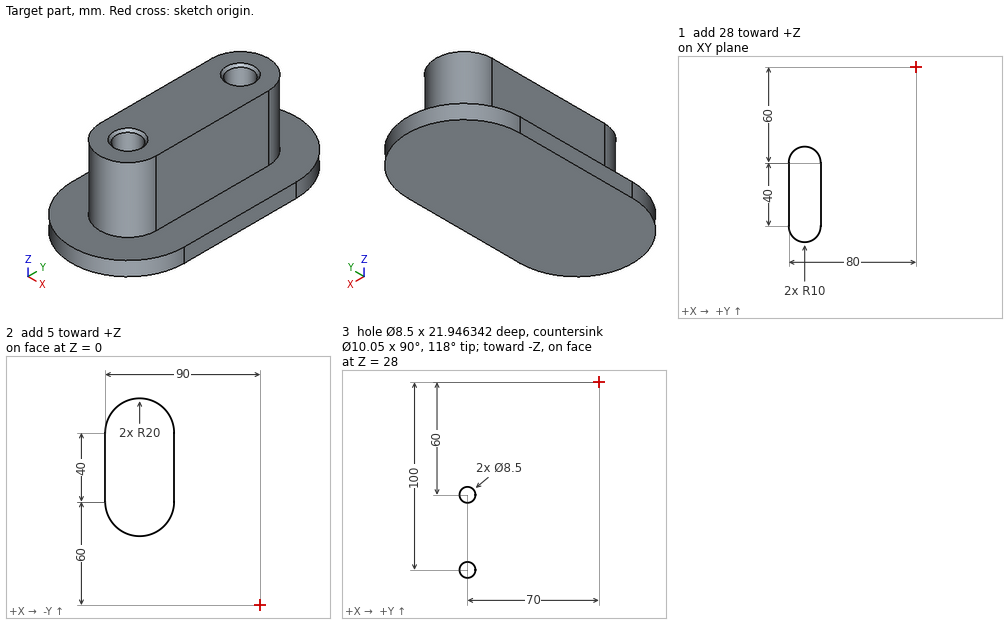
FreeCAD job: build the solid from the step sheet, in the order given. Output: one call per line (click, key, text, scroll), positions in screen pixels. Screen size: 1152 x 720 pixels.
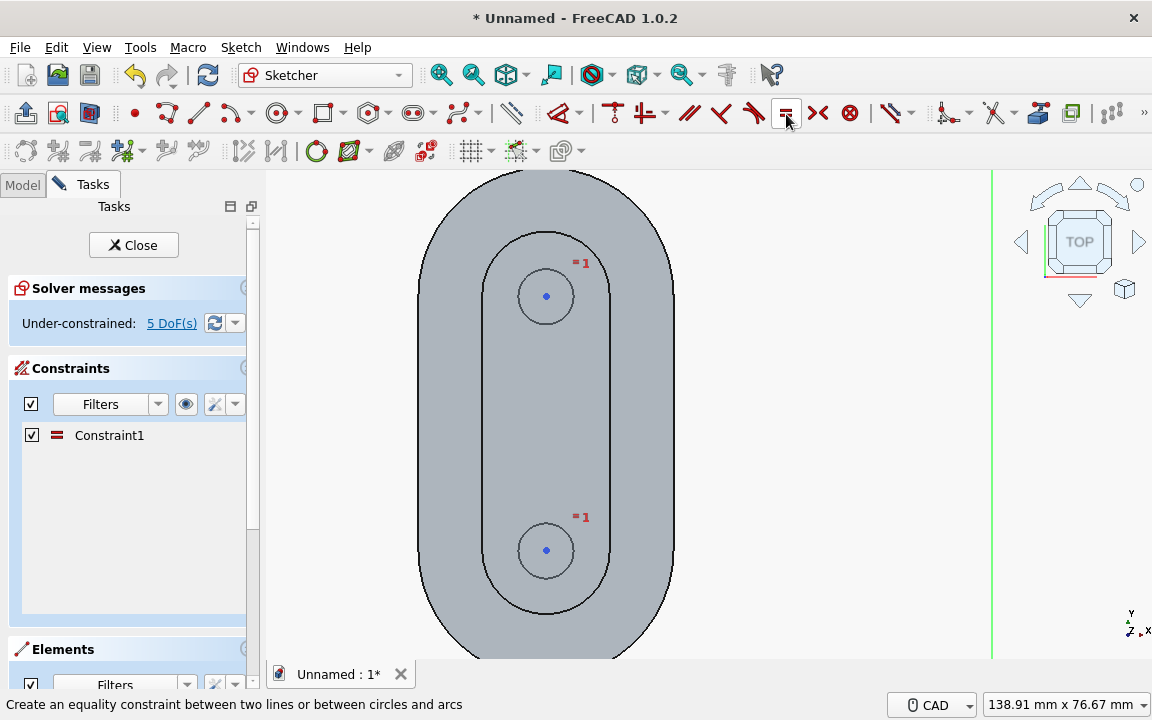
click(546, 297)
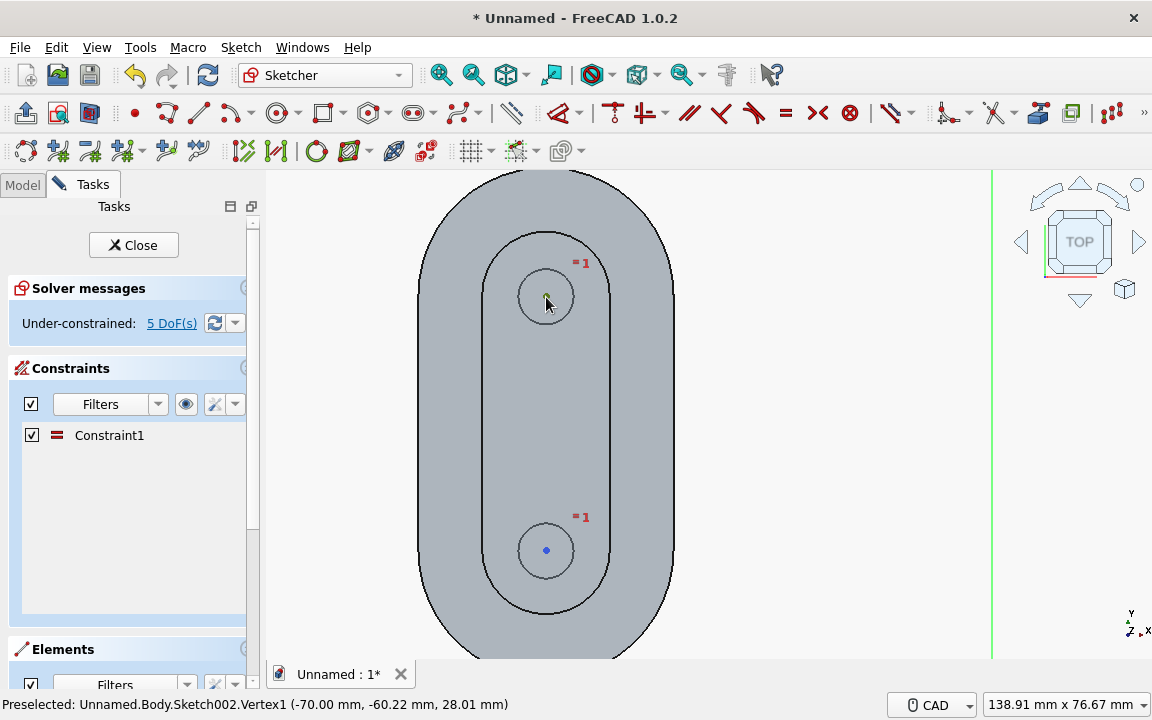
click(546, 551)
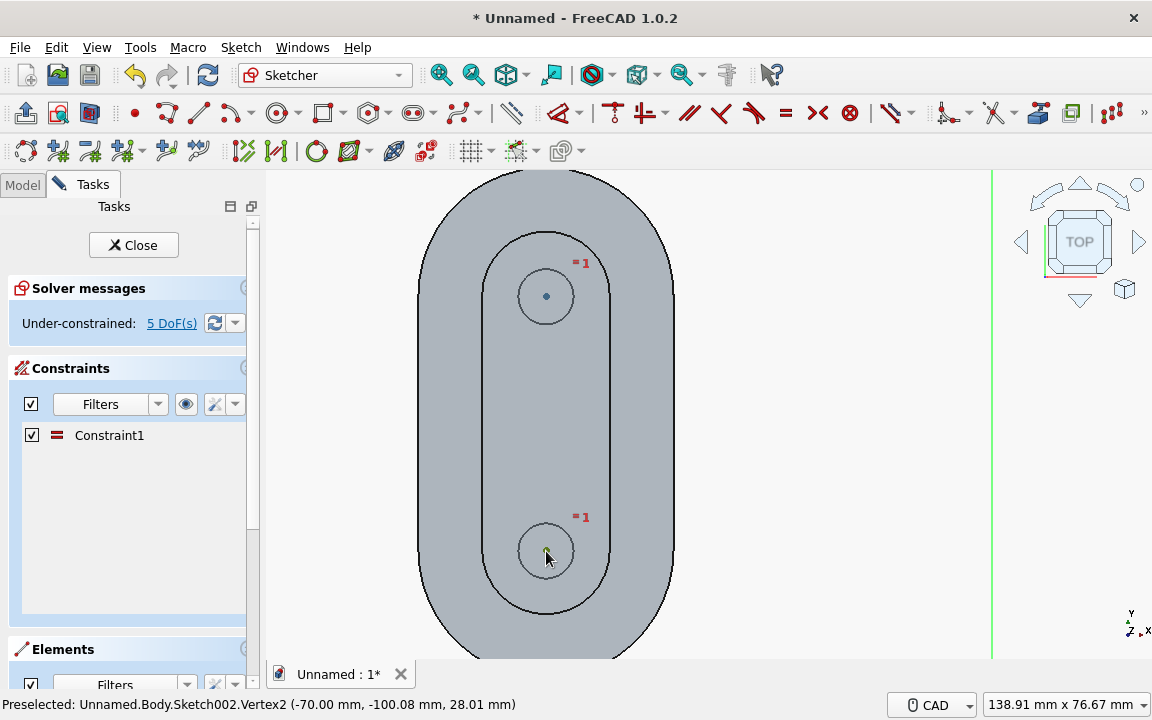
click(668, 114)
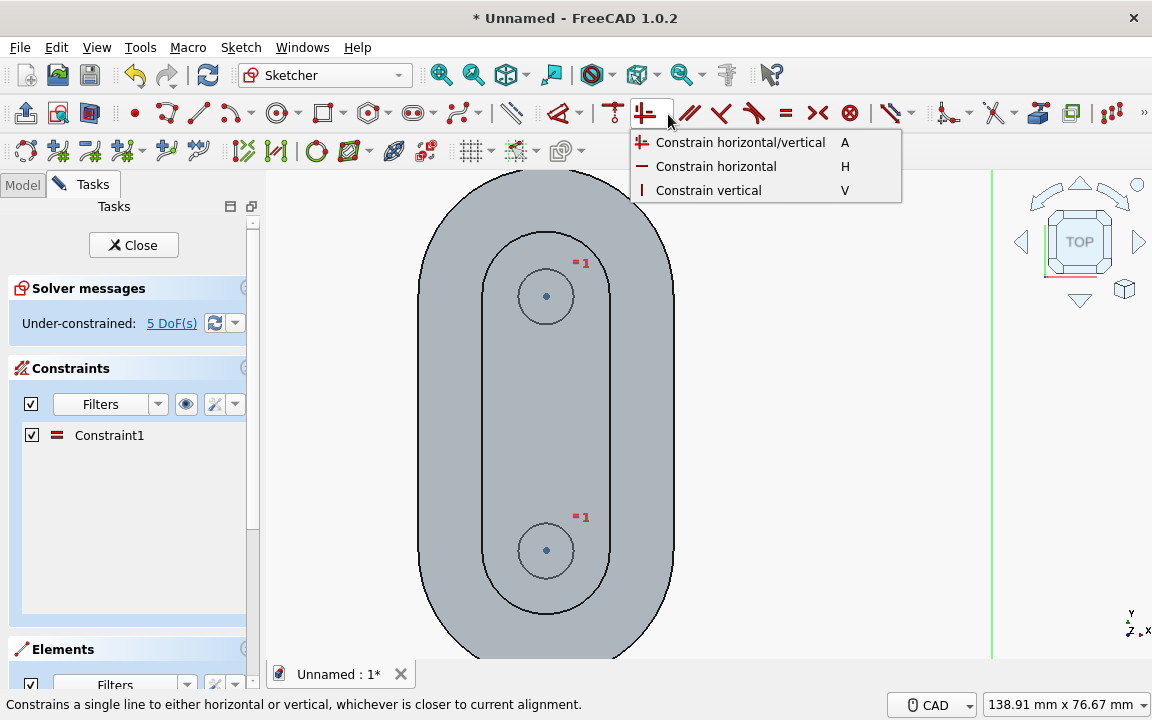
click(766, 190)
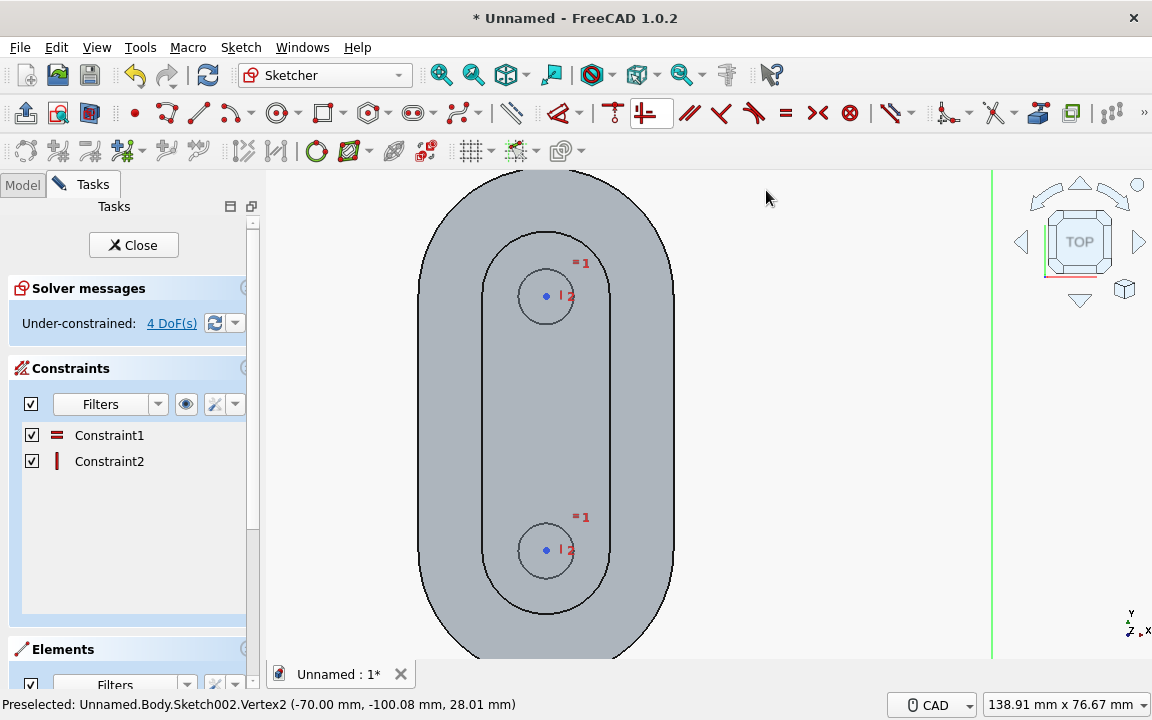
click(558, 114)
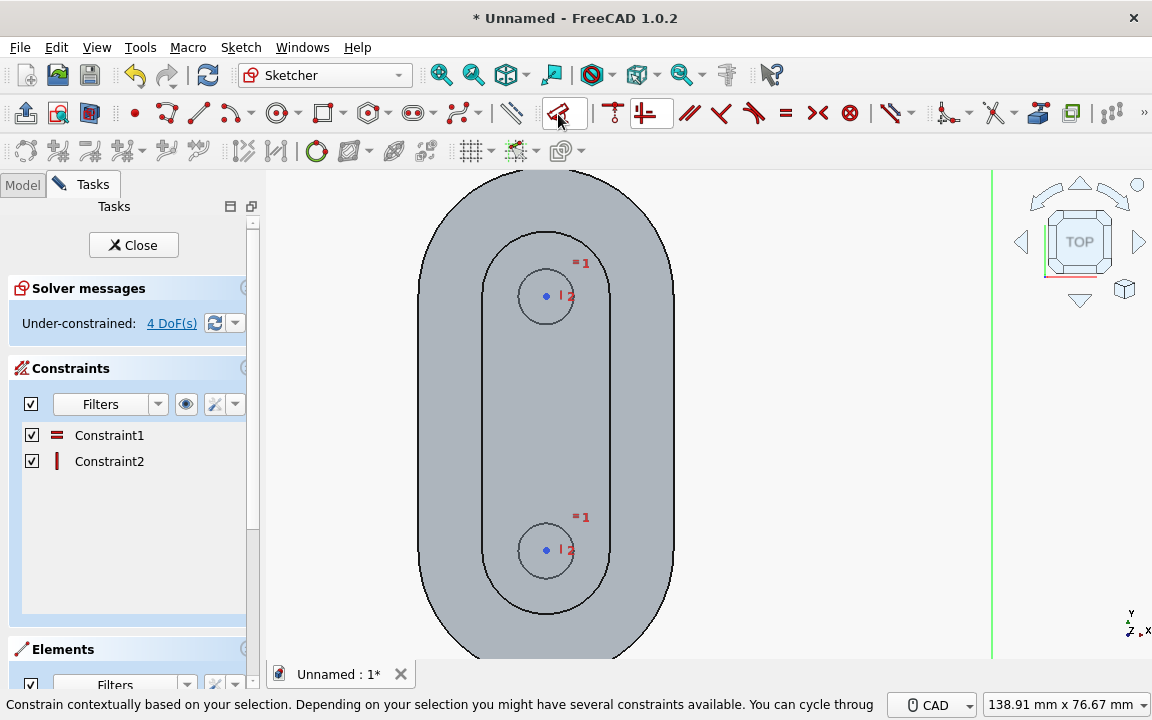
click(565, 277)
click(587, 254)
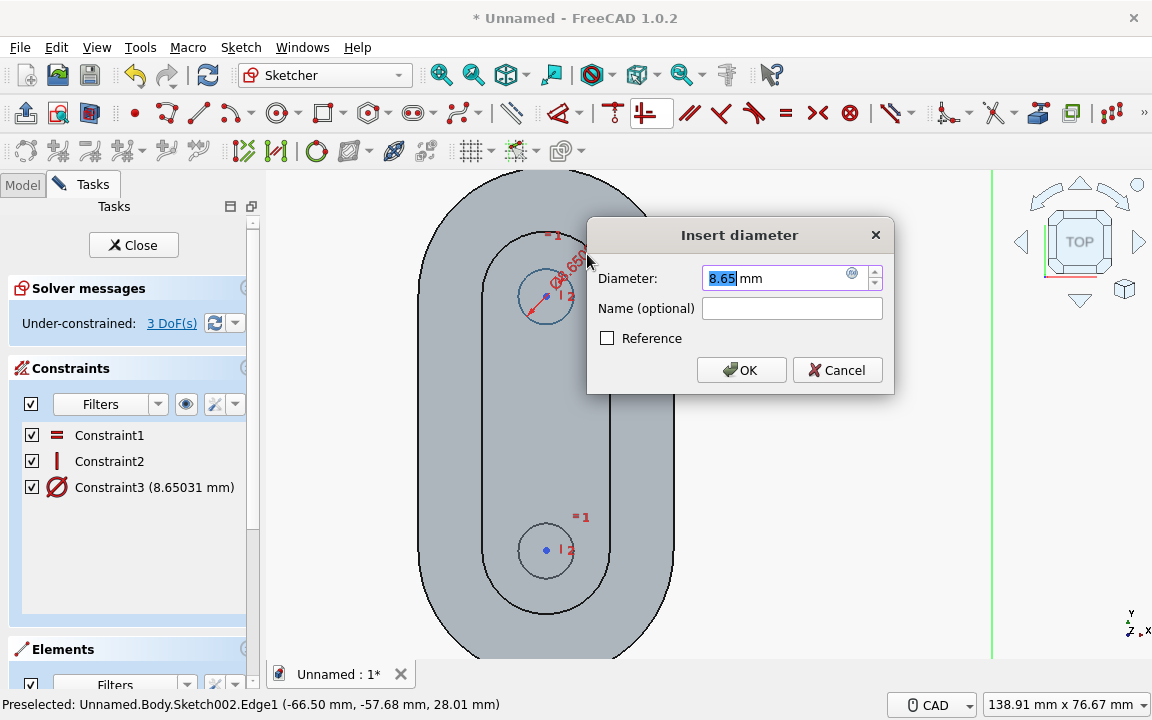
text(8.5)
key(Return)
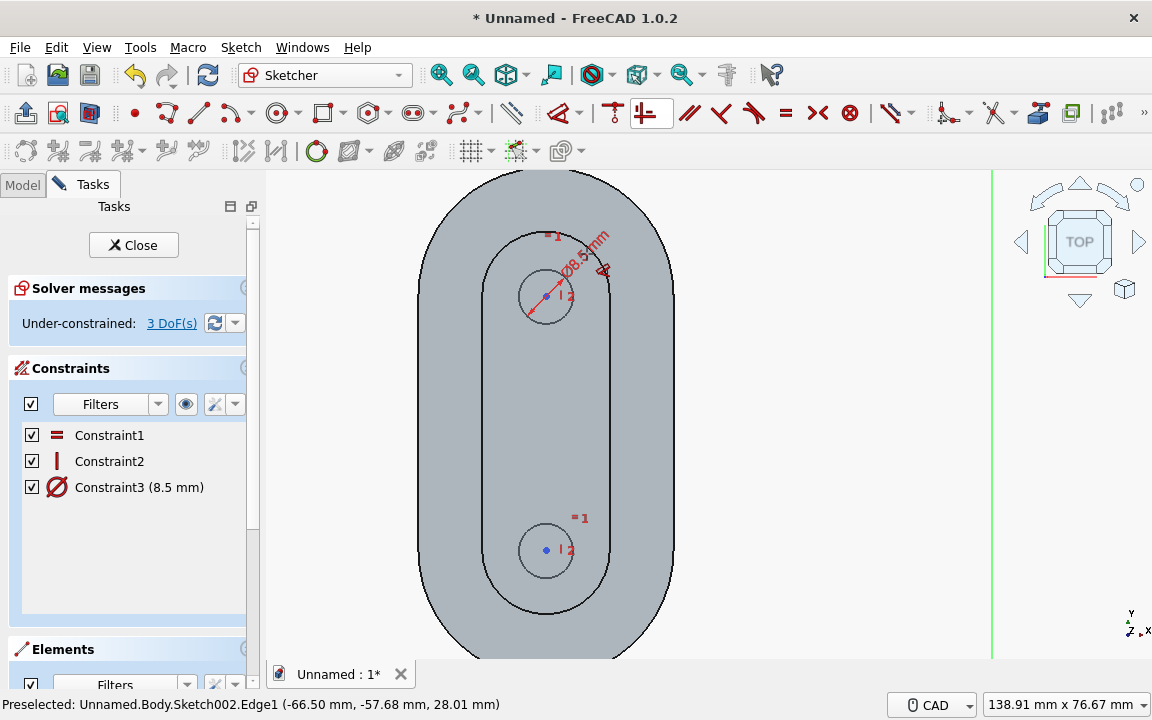
click(546, 297)
click(767, 331)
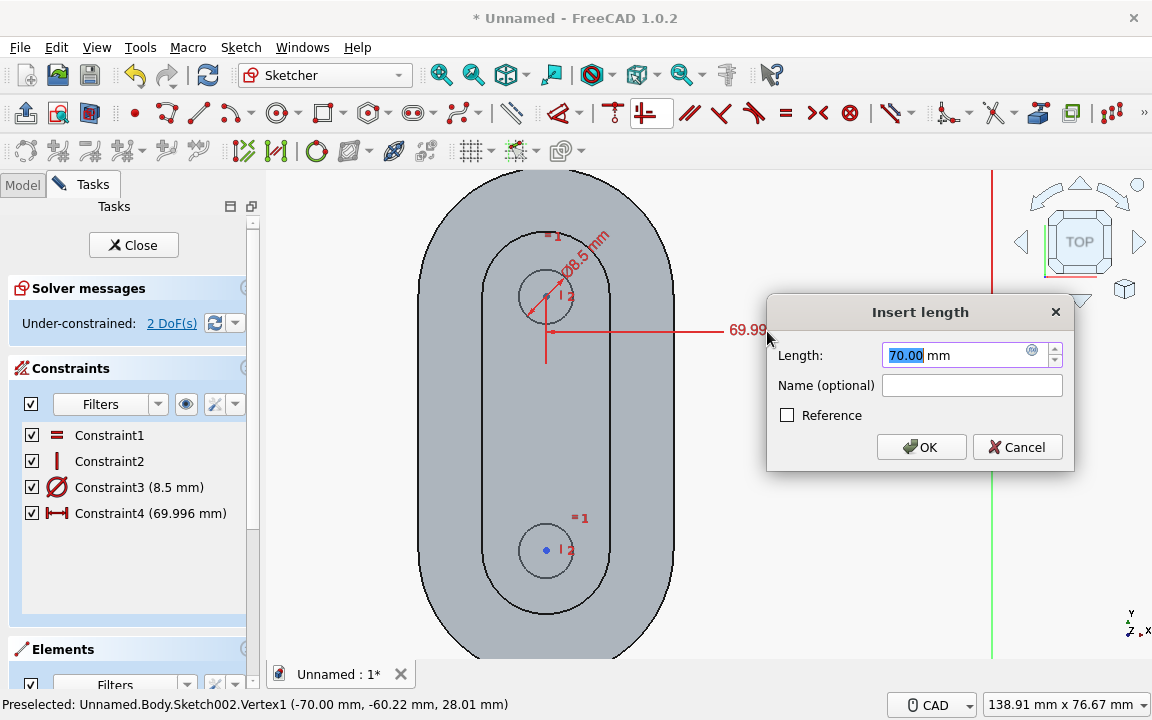
text(70)
key(Return)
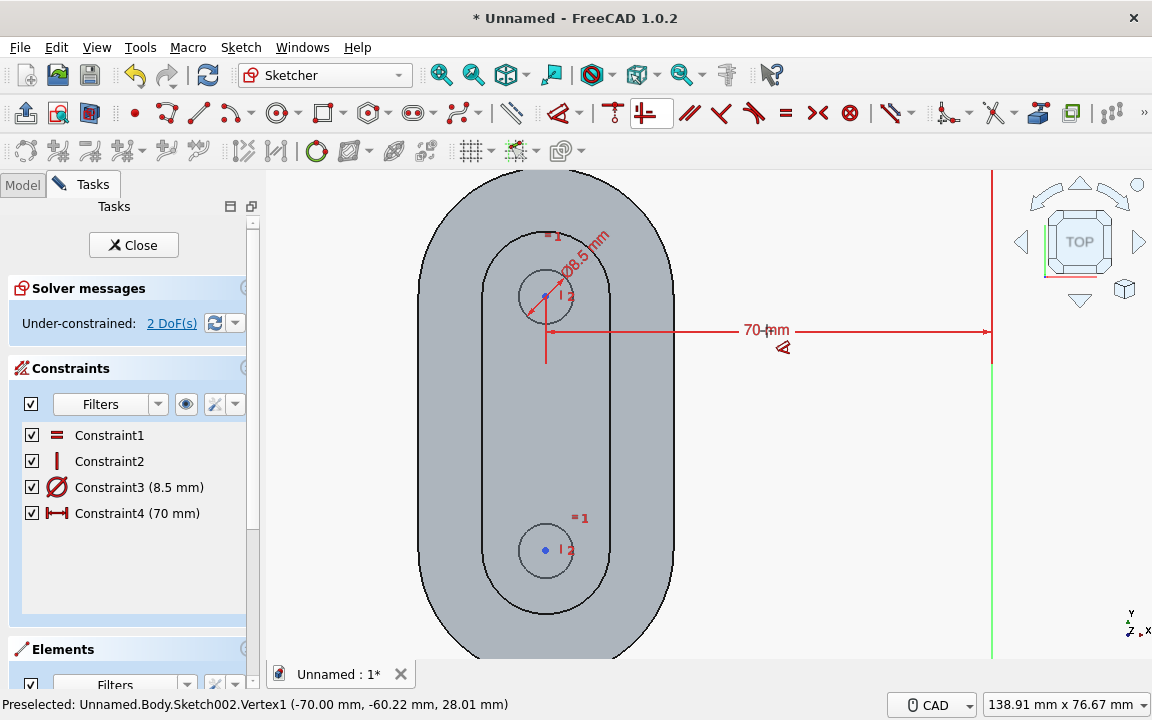
click(546, 297)
click(512, 247)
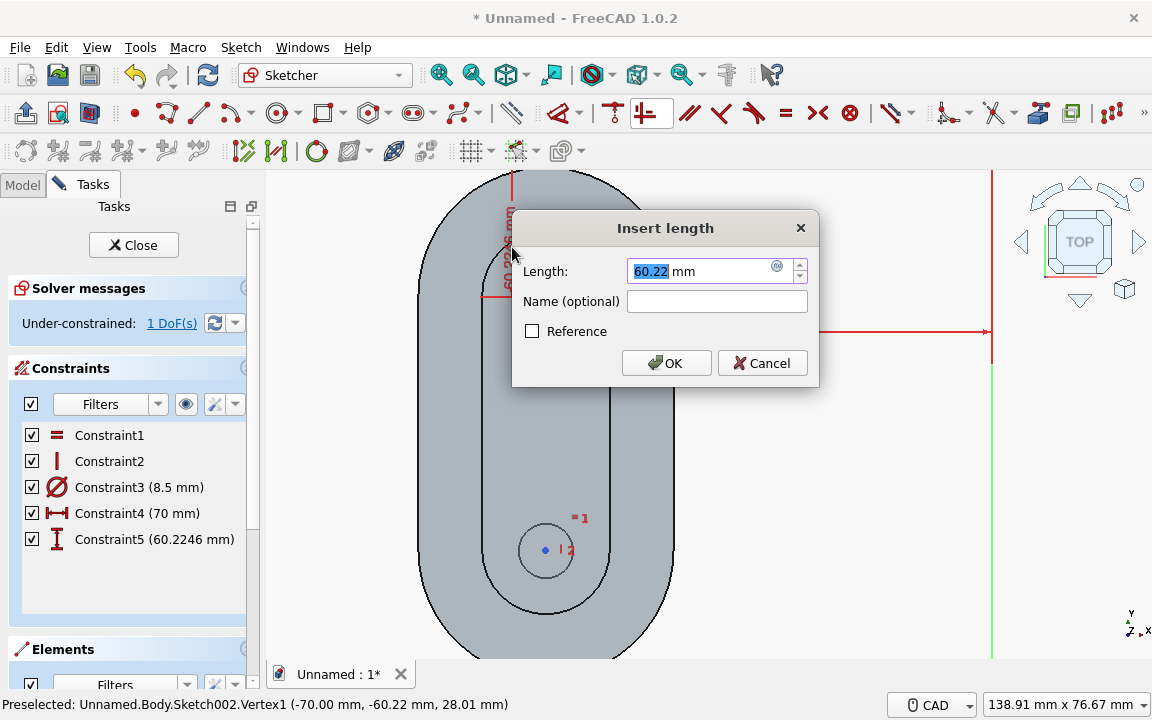
text(60)
key(Return)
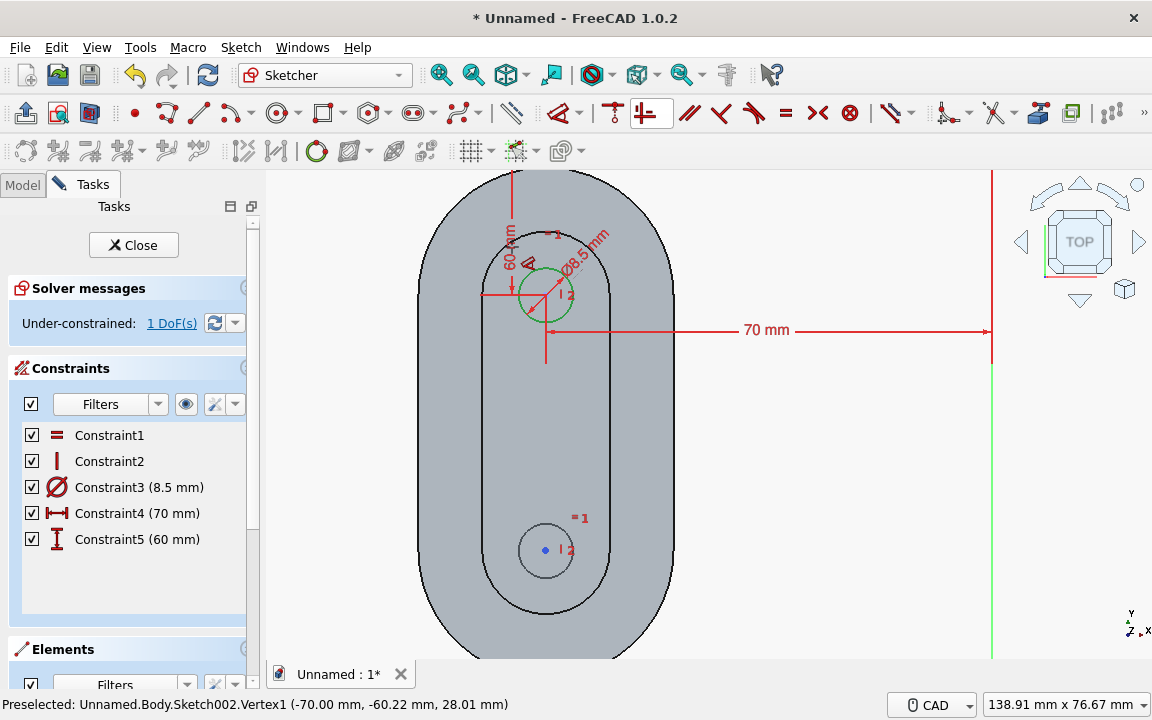
click(546, 551)
click(512, 374)